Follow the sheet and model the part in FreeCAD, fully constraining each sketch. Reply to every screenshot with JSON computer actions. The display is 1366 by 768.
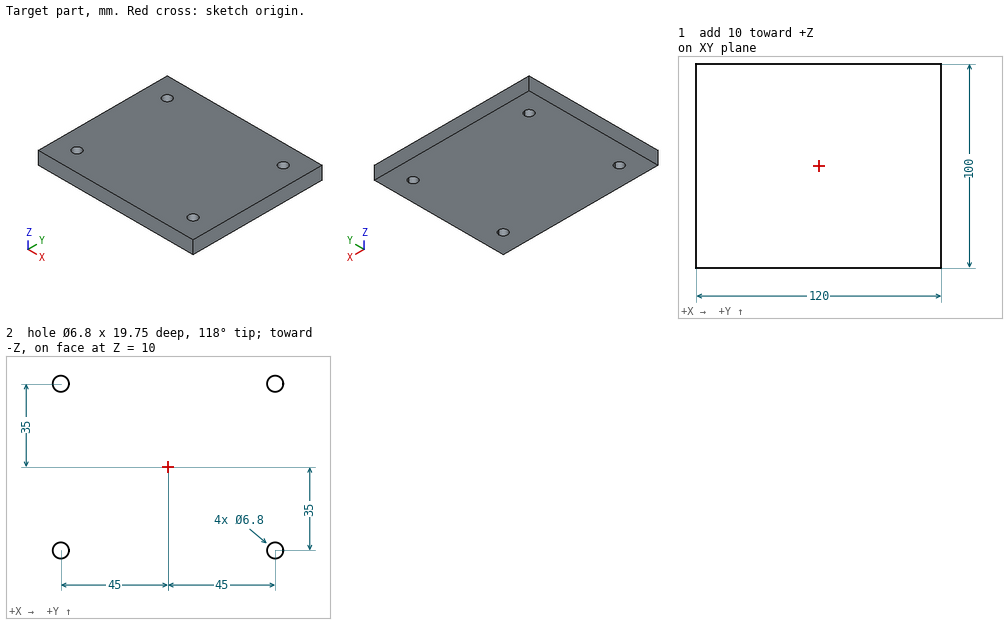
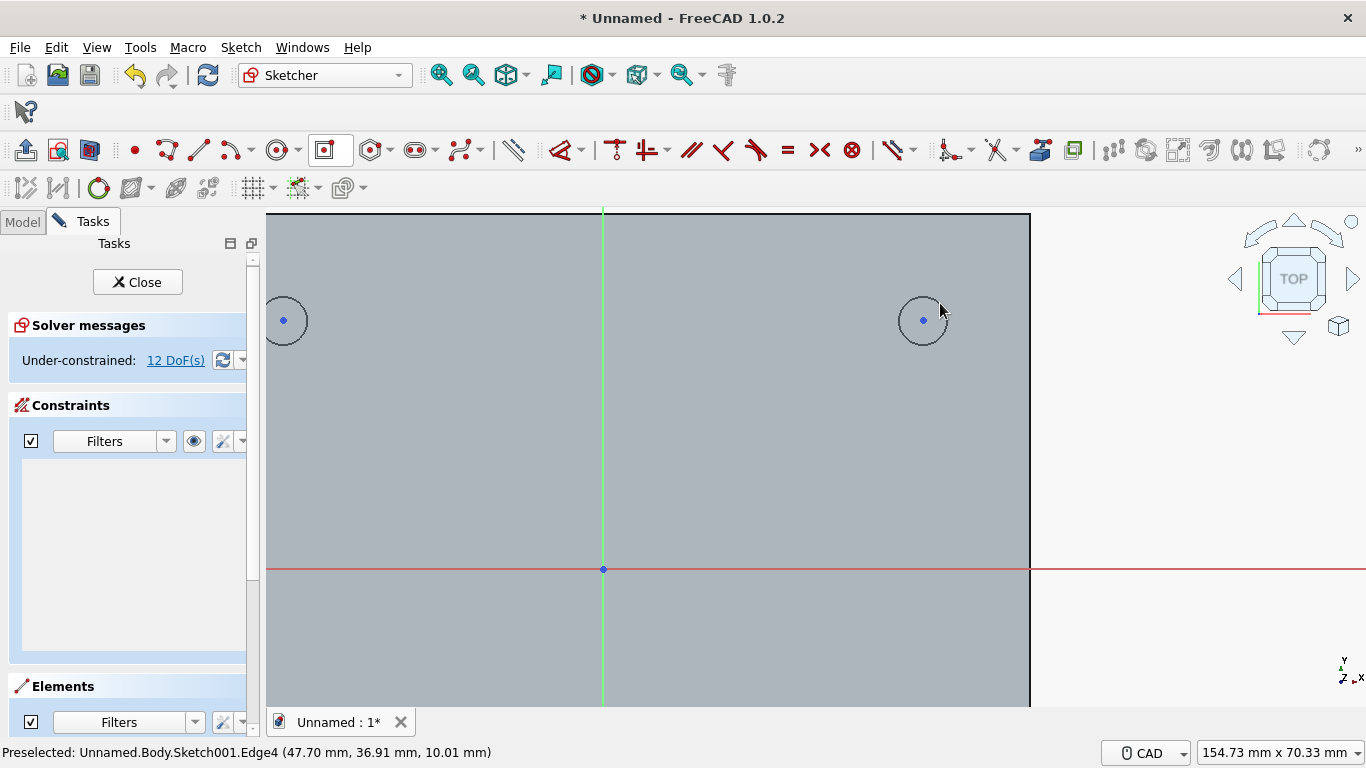
{"action": "scroll", "coordinate": [923, 320], "scroll_direction": "down", "scroll_amount": 3}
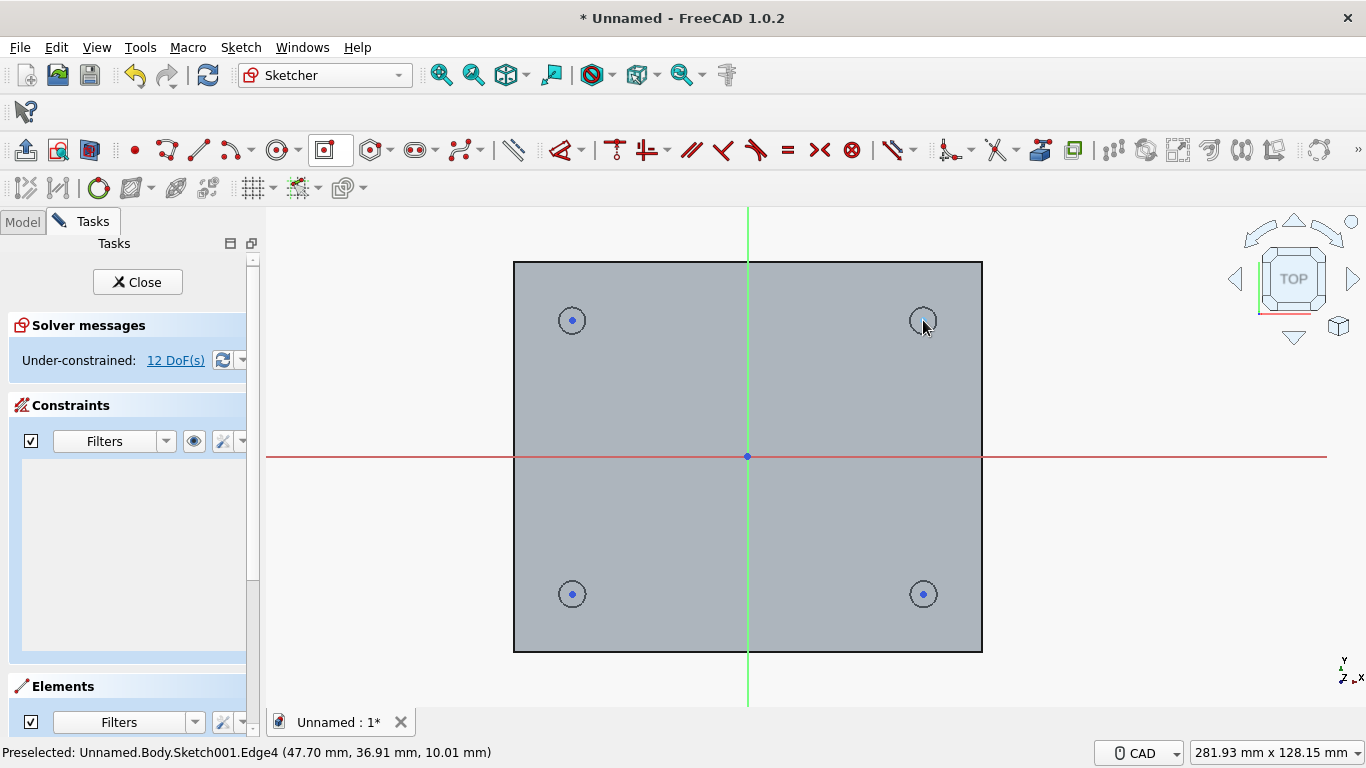
{"action": "left_click", "coordinate": [933, 585]}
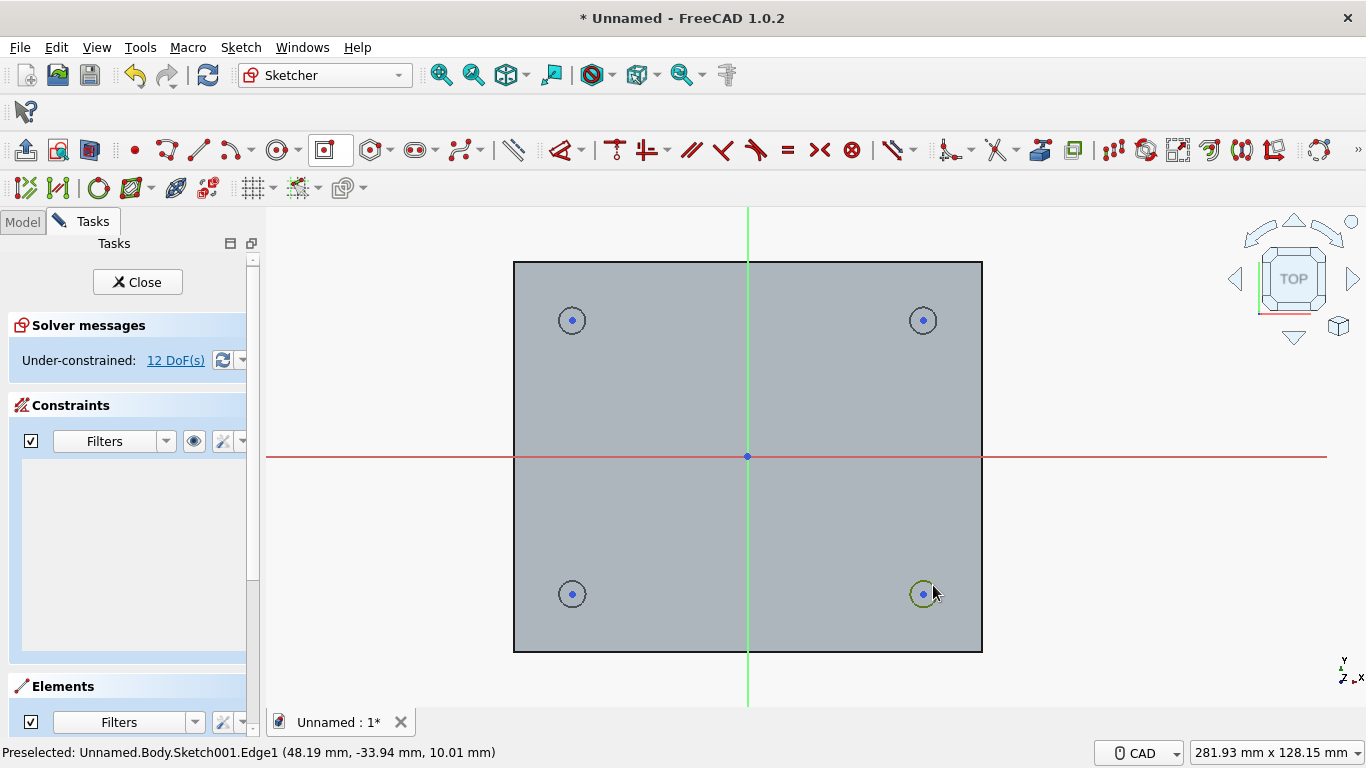
{"action": "left_click", "coordinate": [582, 585]}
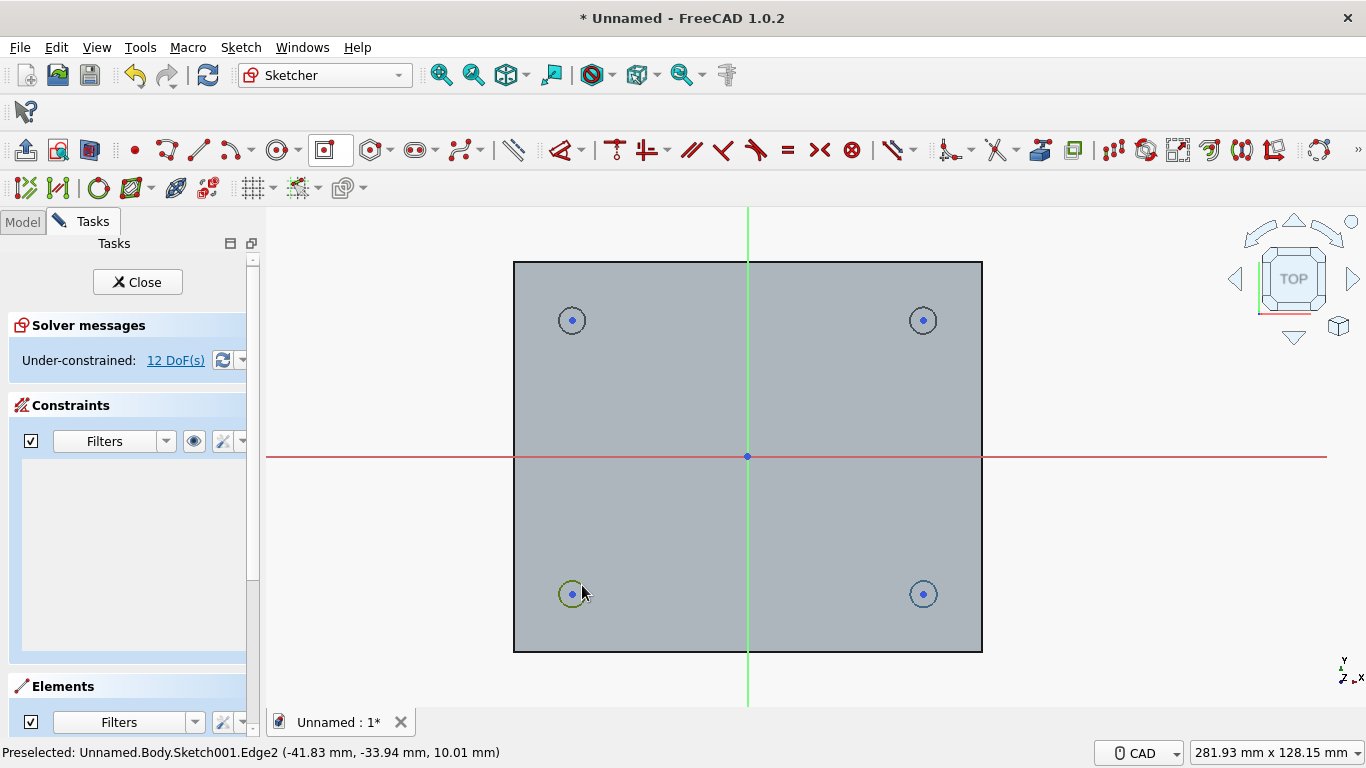
{"action": "left_click", "coordinate": [581, 311]}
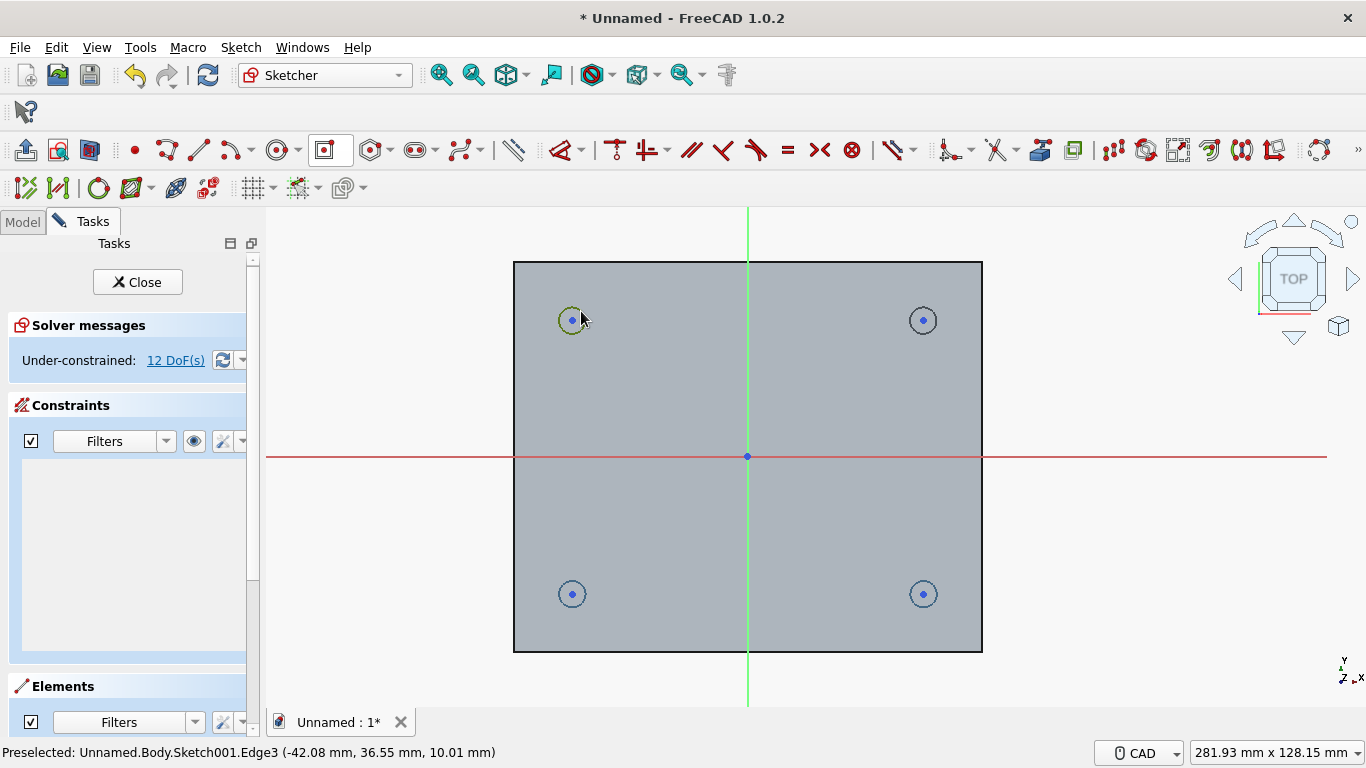
{"action": "left_click", "coordinate": [933, 311]}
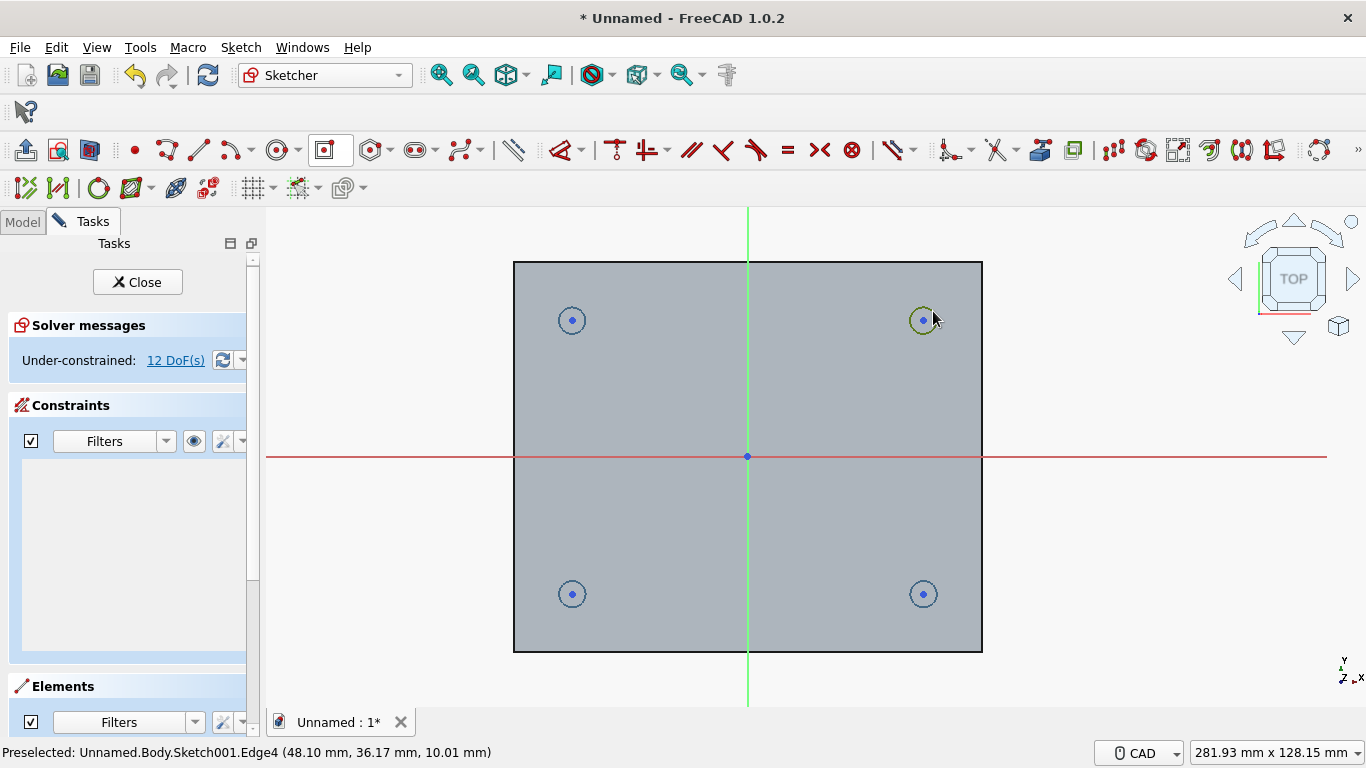
{"action": "left_click", "coordinate": [788, 150]}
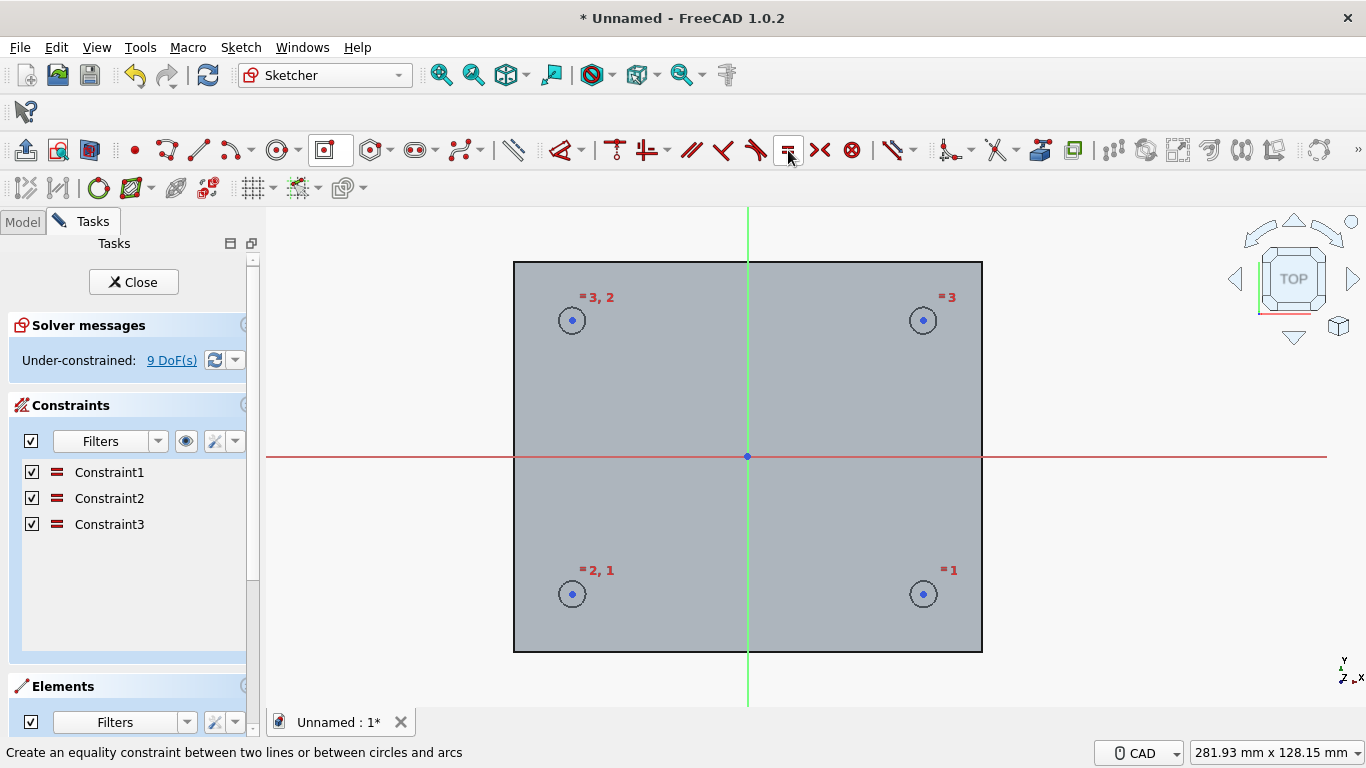
{"action": "left_click", "coordinate": [924, 594]}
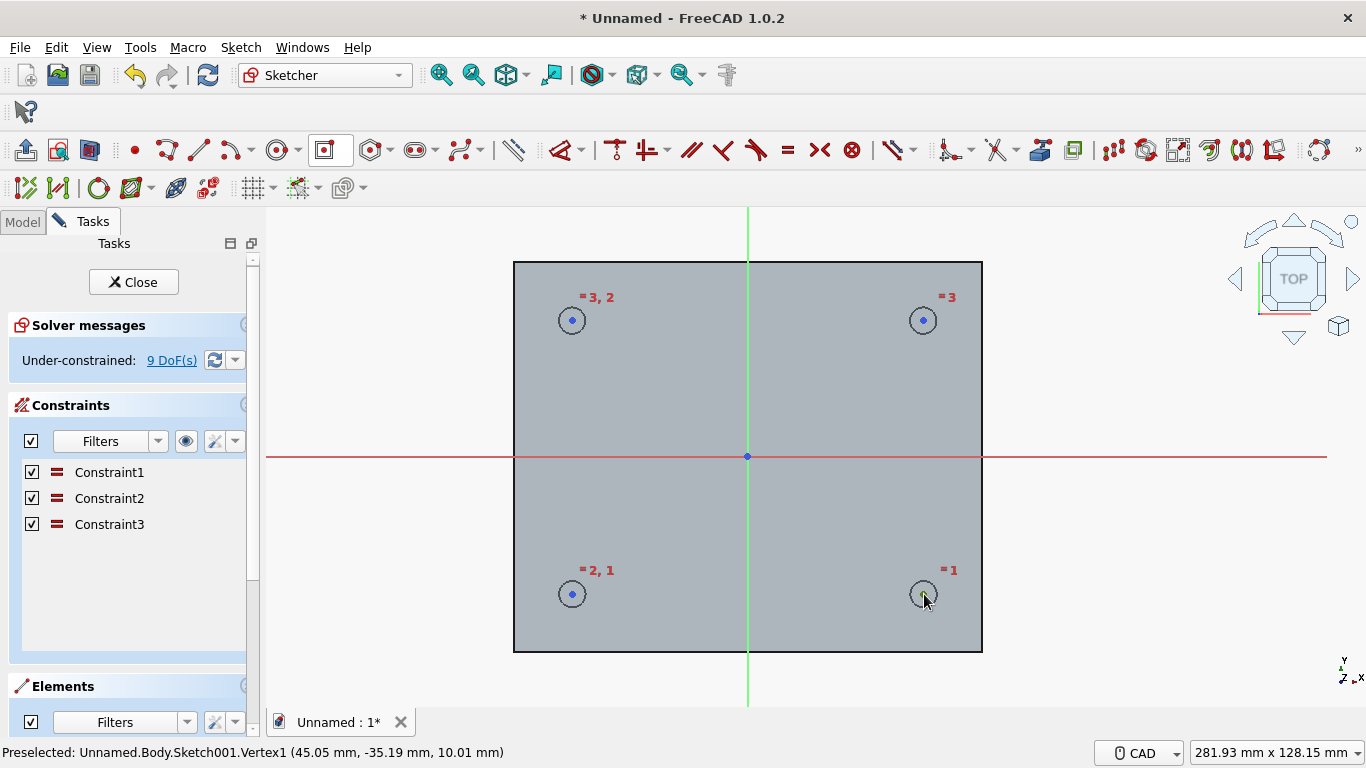
{"action": "left_click", "coordinate": [572, 594]}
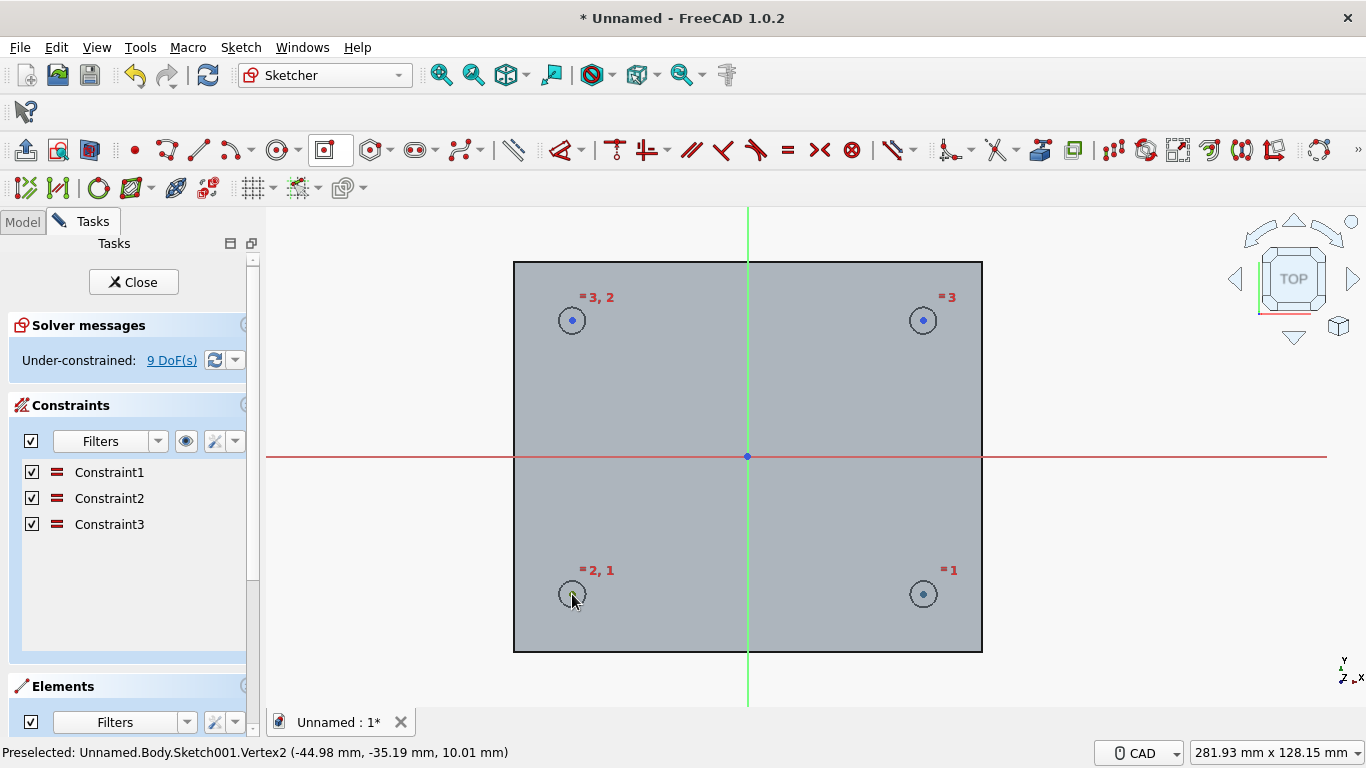
{"action": "left_click", "coordinate": [670, 150]}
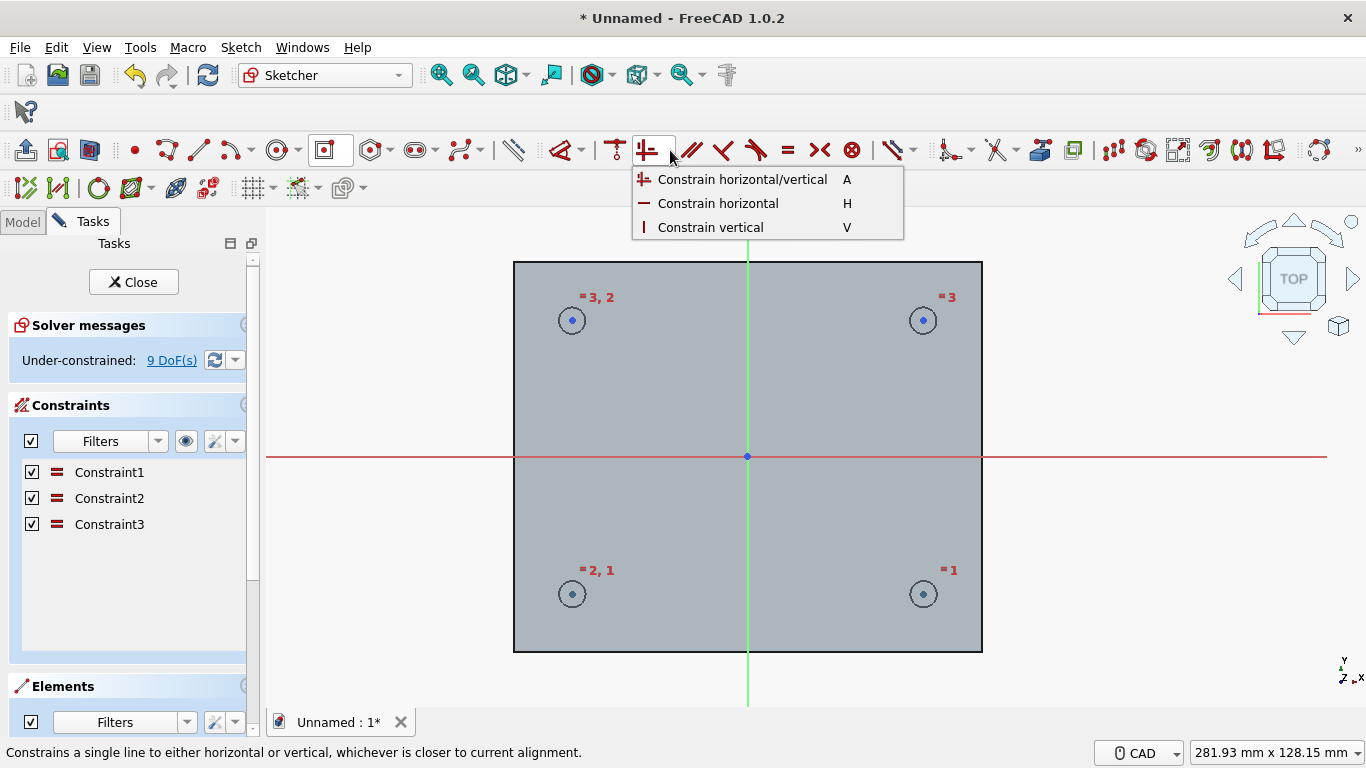
{"action": "left_click", "coordinate": [768, 203]}